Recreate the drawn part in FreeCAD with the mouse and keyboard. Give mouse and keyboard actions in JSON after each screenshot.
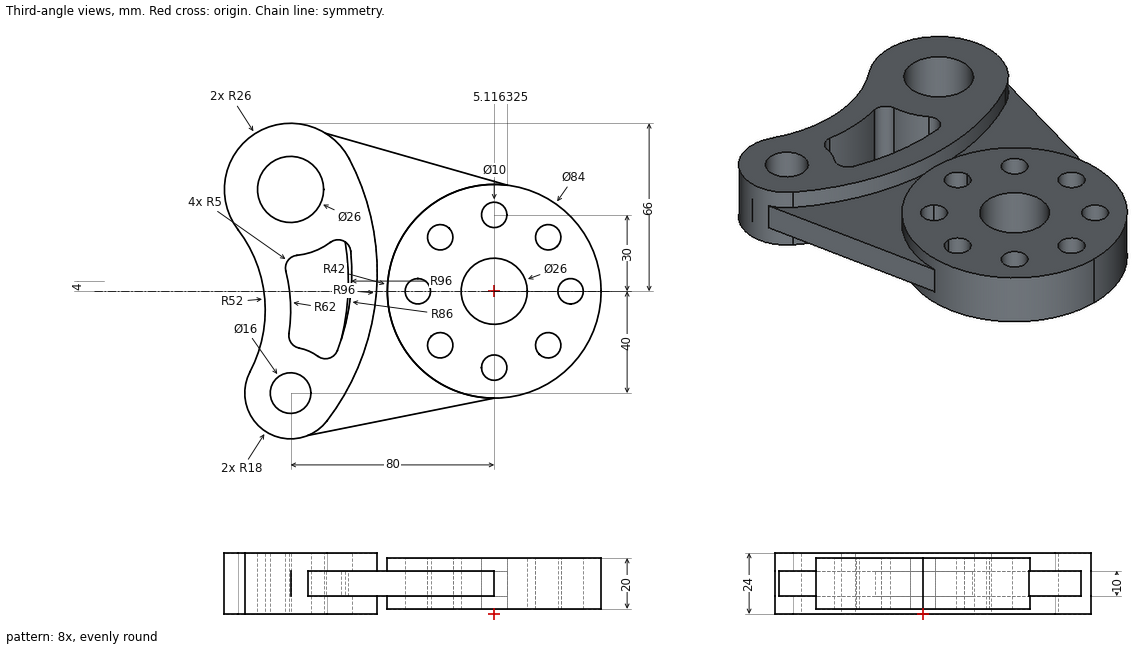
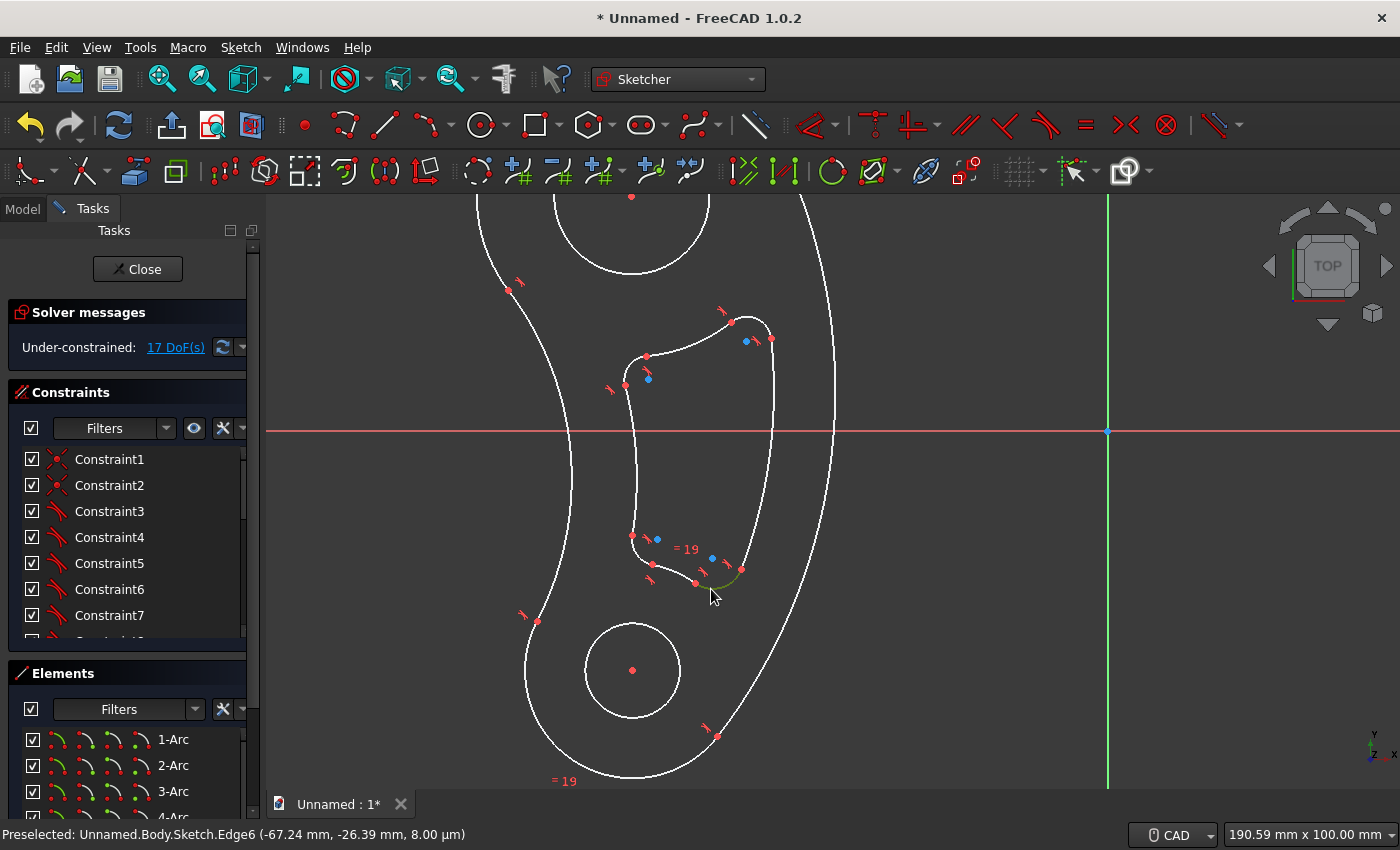
{"action": "left_click", "coordinate": [633, 548]}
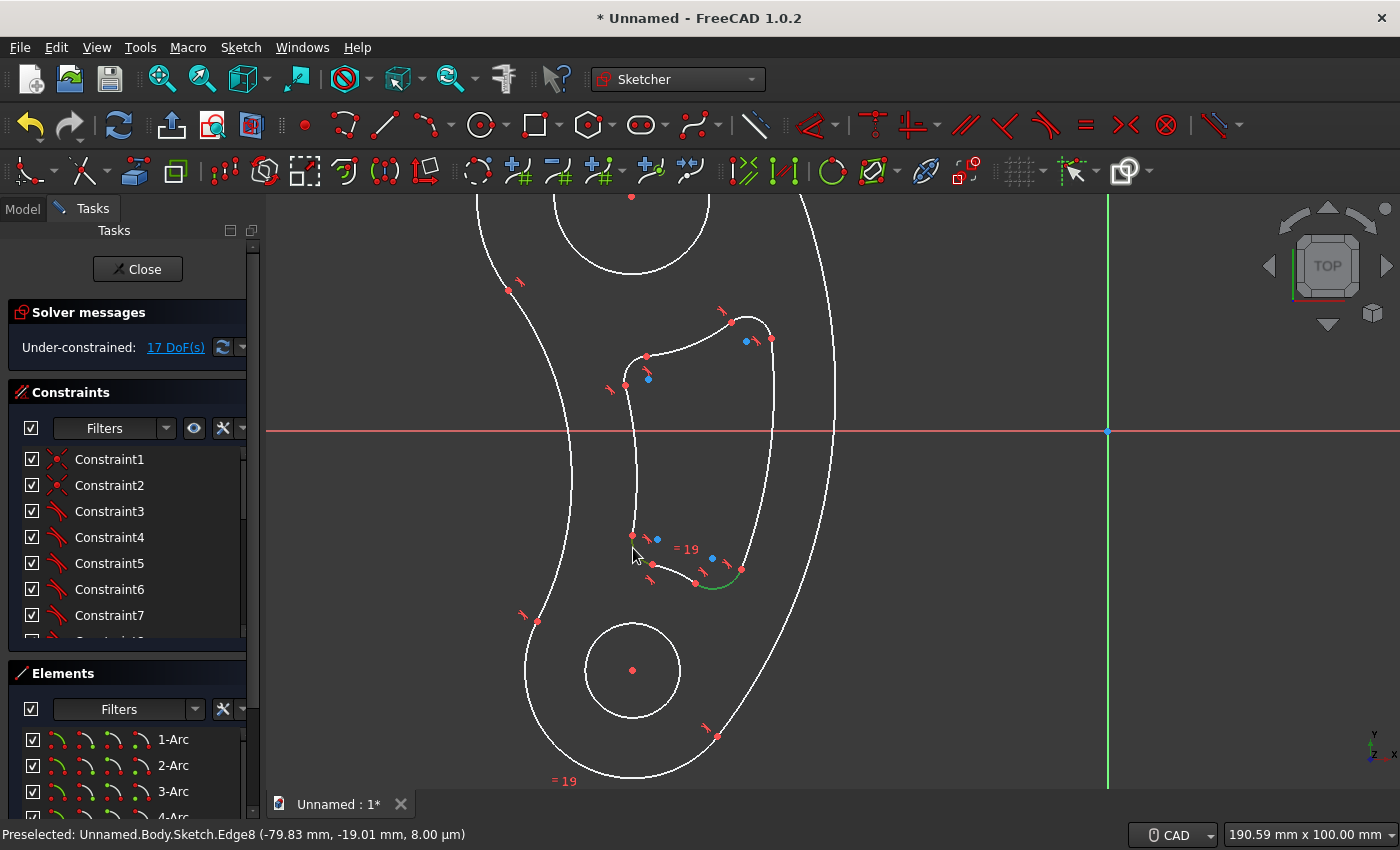
{"action": "left_click", "coordinate": [635, 360]}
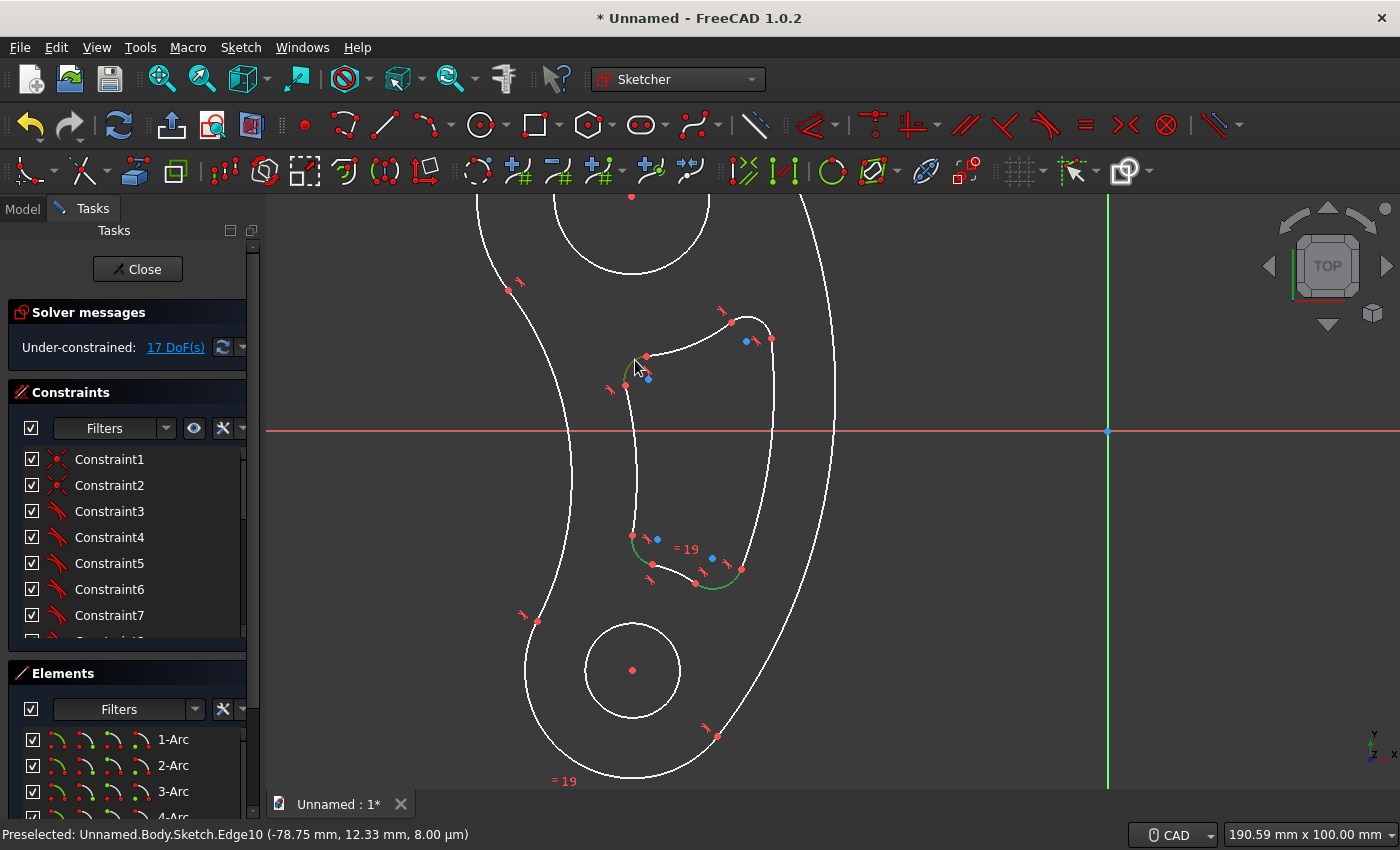
{"action": "left_click", "coordinate": [765, 325]}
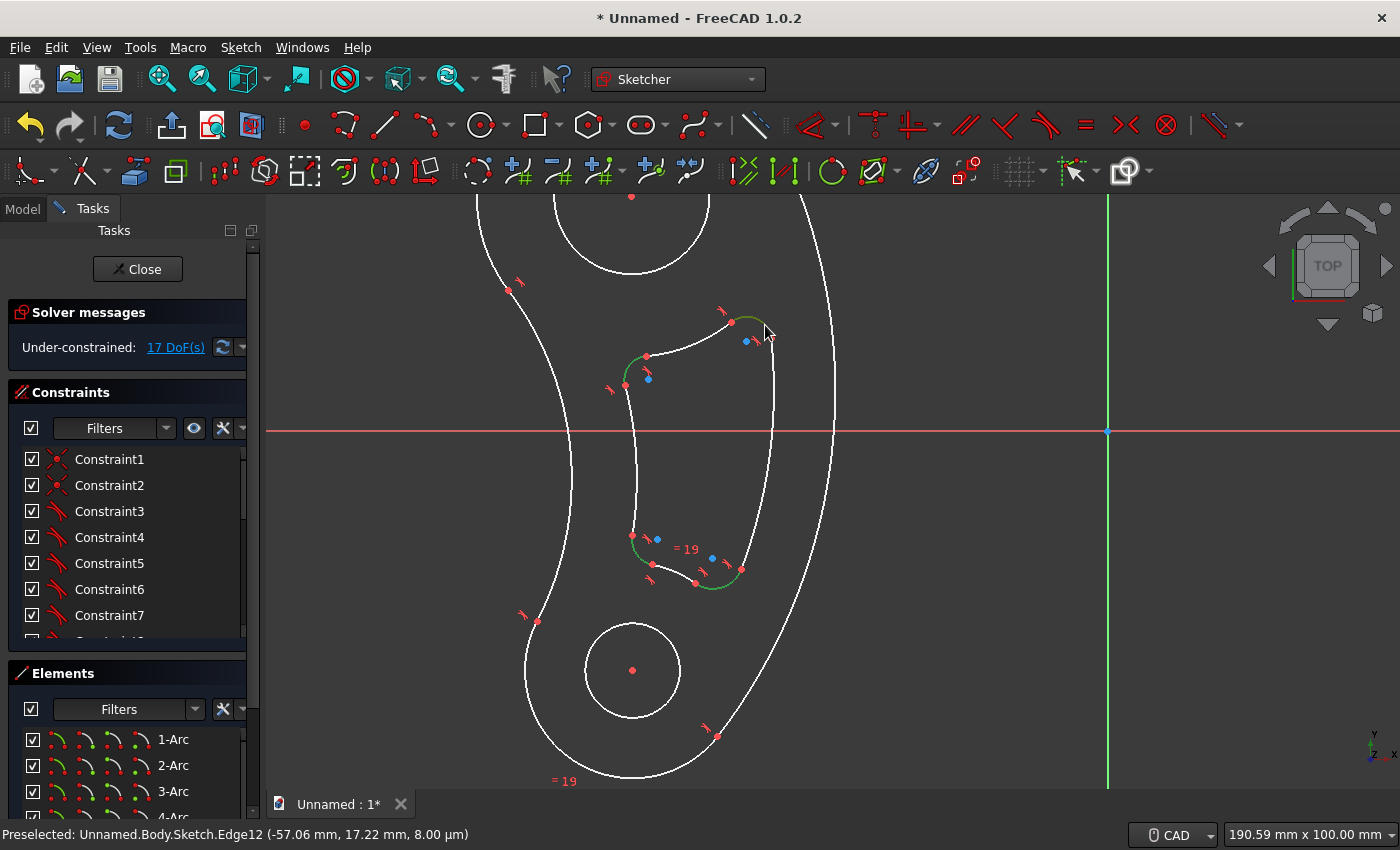
{"action": "left_click", "coordinate": [1086, 126]}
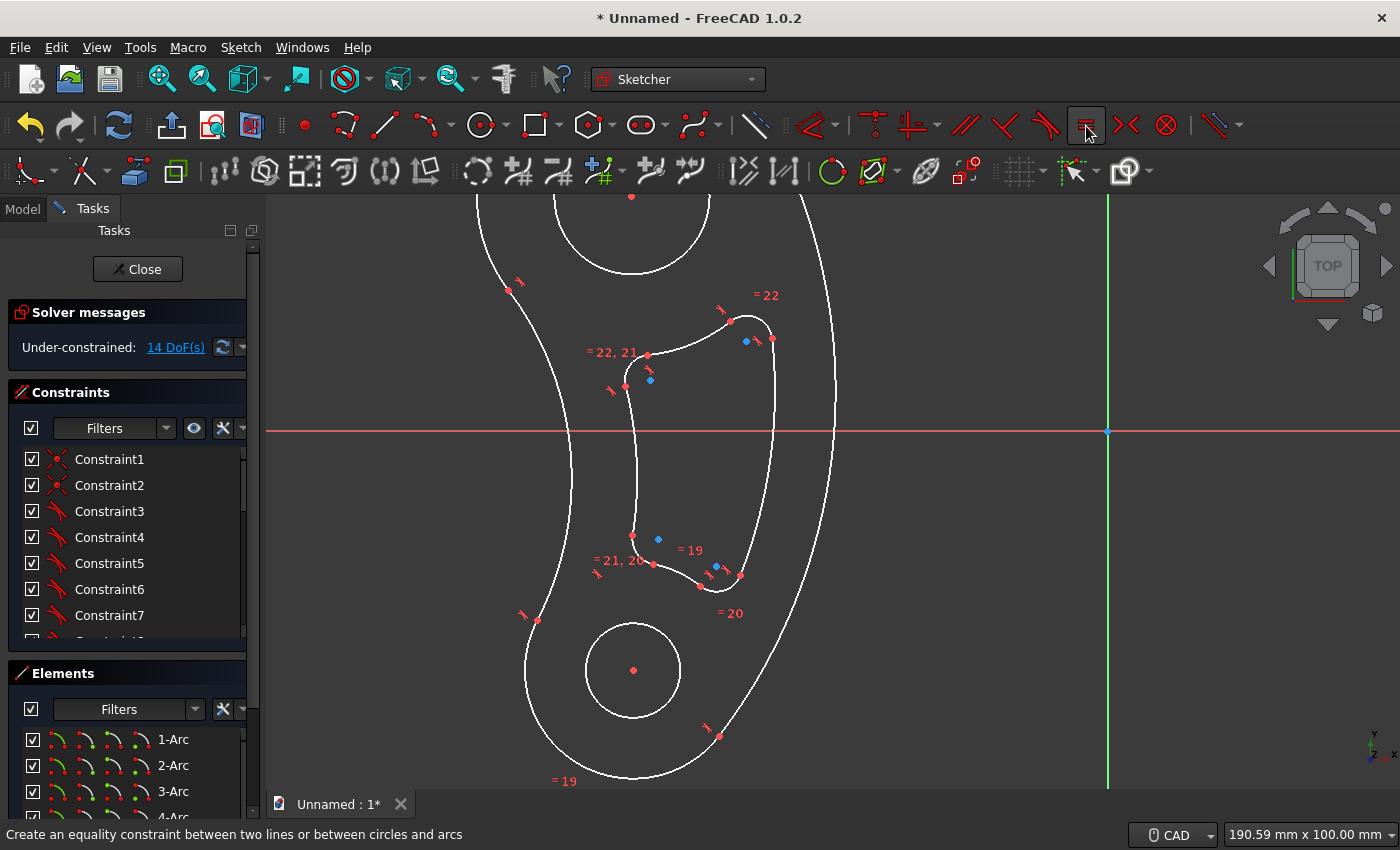
{"action": "scroll", "coordinate": [711, 589], "scroll_direction": "down", "scroll_amount": 3}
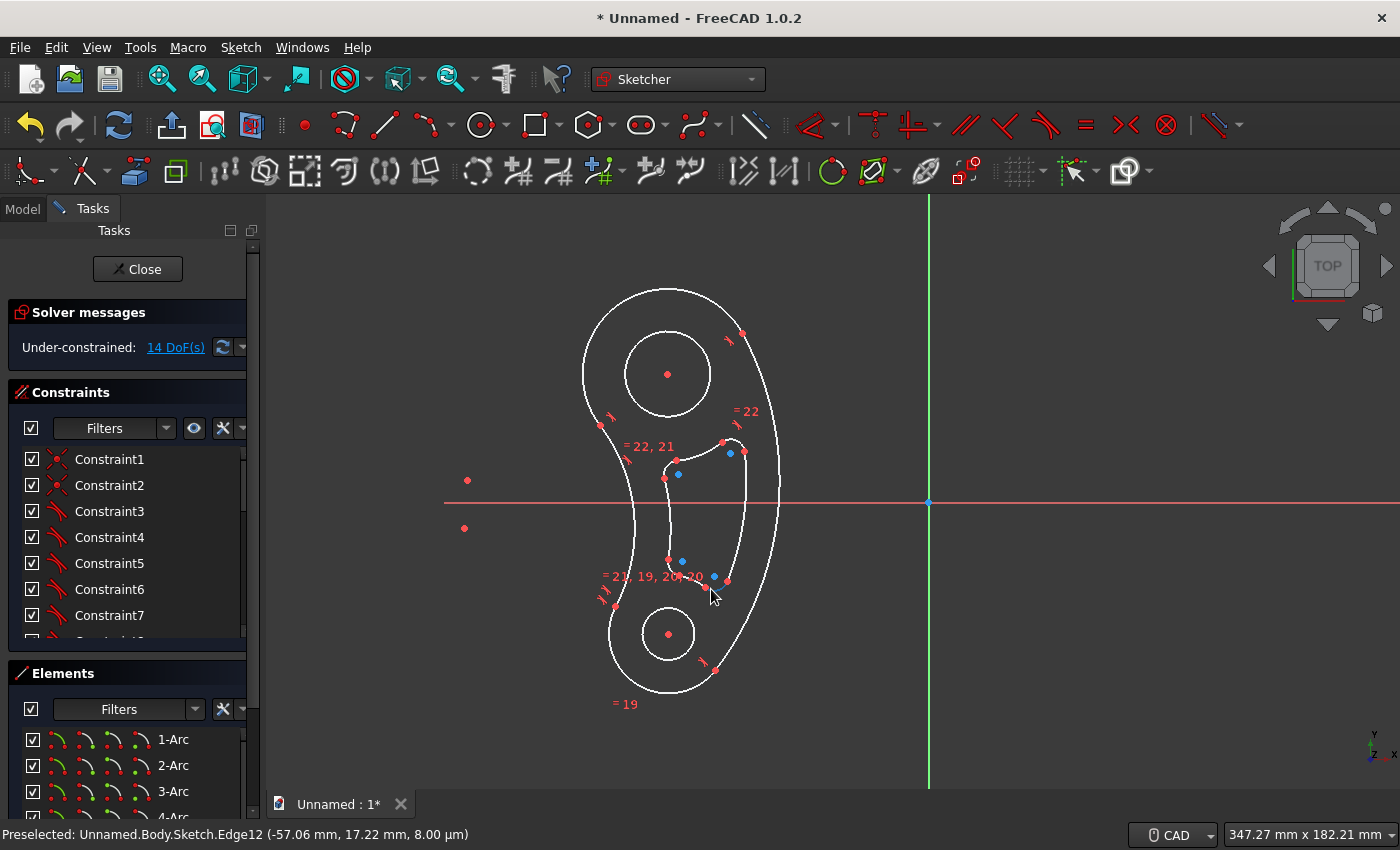
{"action": "left_click", "coordinate": [675, 289]}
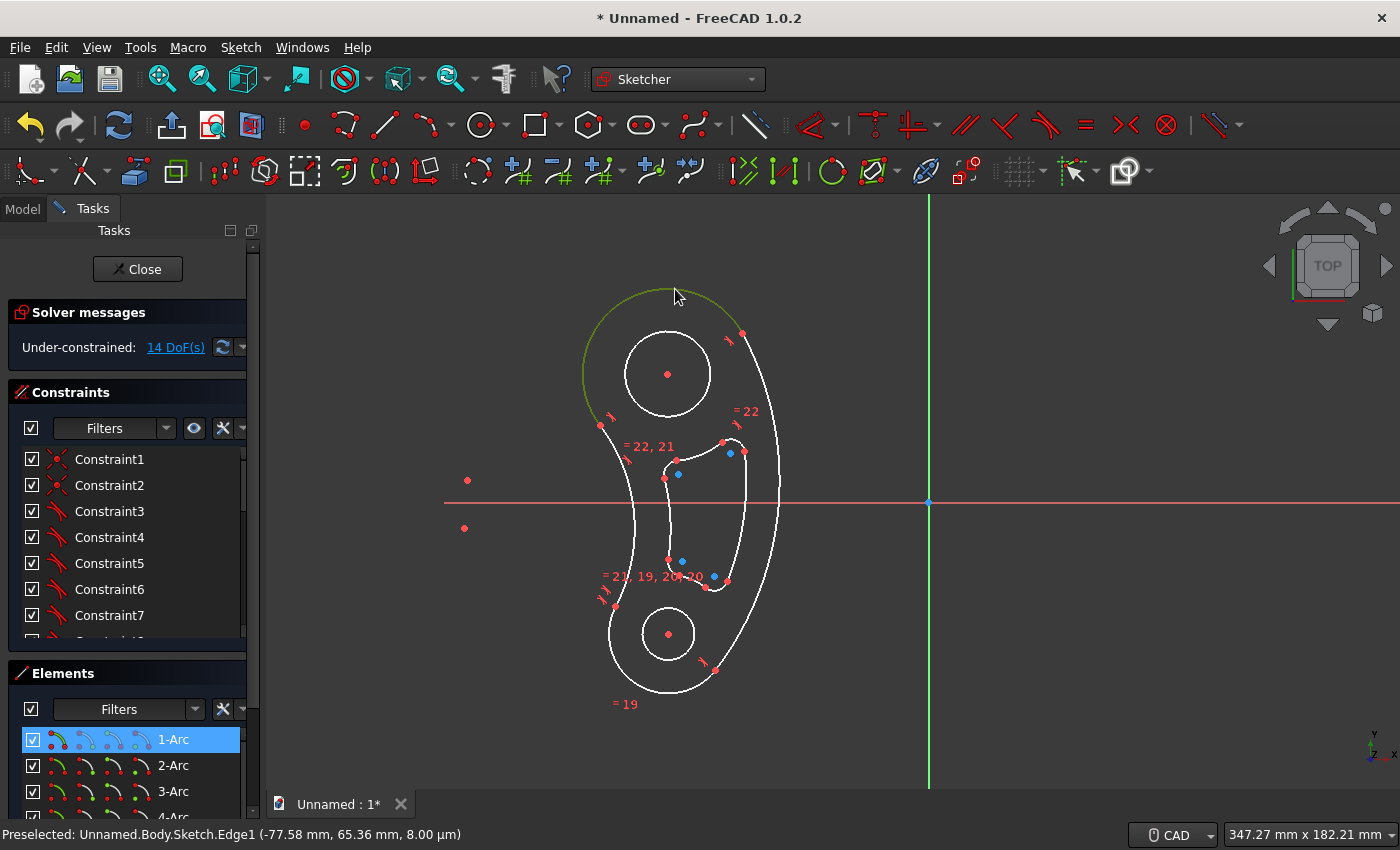
{"action": "left_click", "coordinate": [691, 458]}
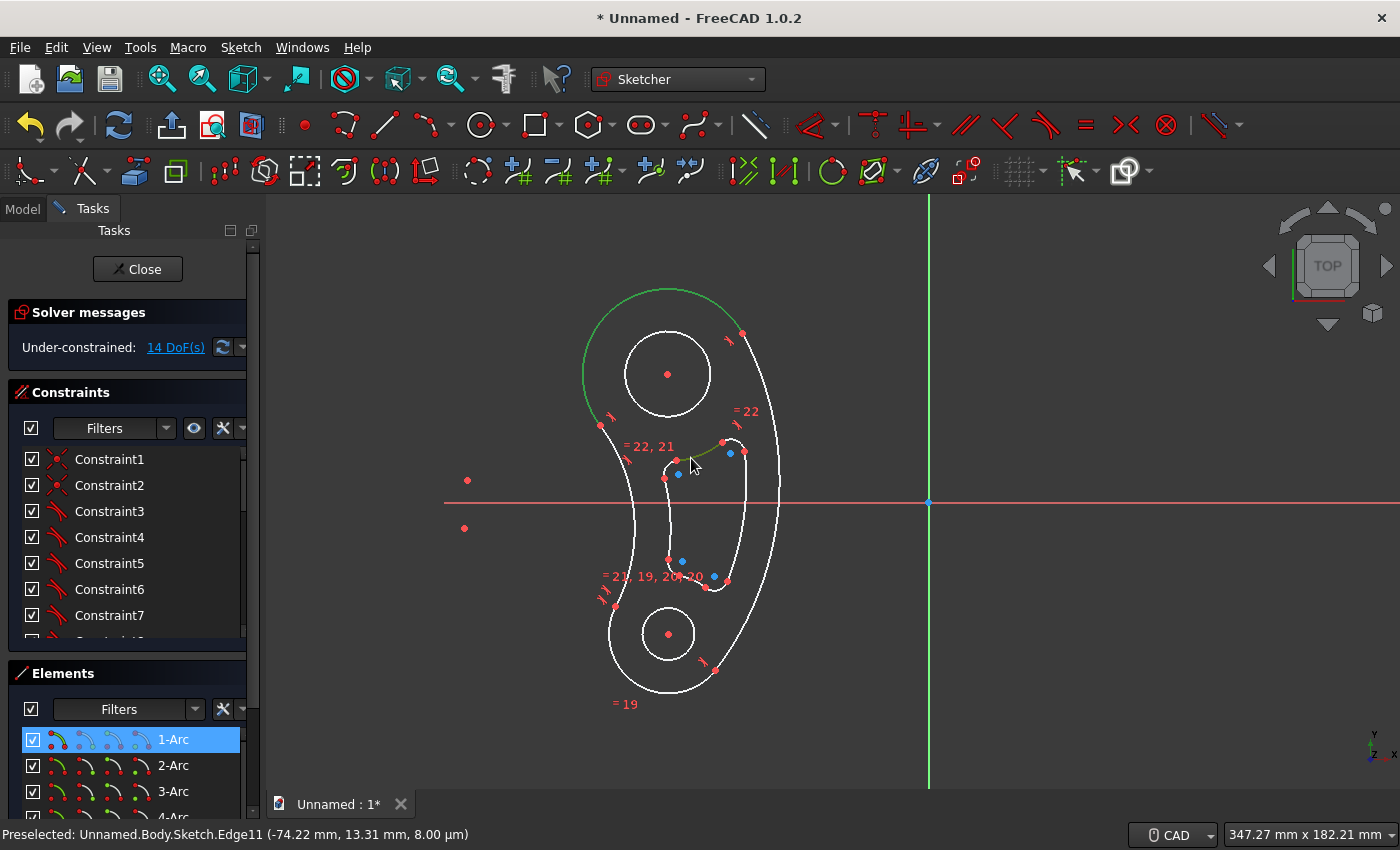
{"action": "left_click", "coordinate": [1086, 126]}